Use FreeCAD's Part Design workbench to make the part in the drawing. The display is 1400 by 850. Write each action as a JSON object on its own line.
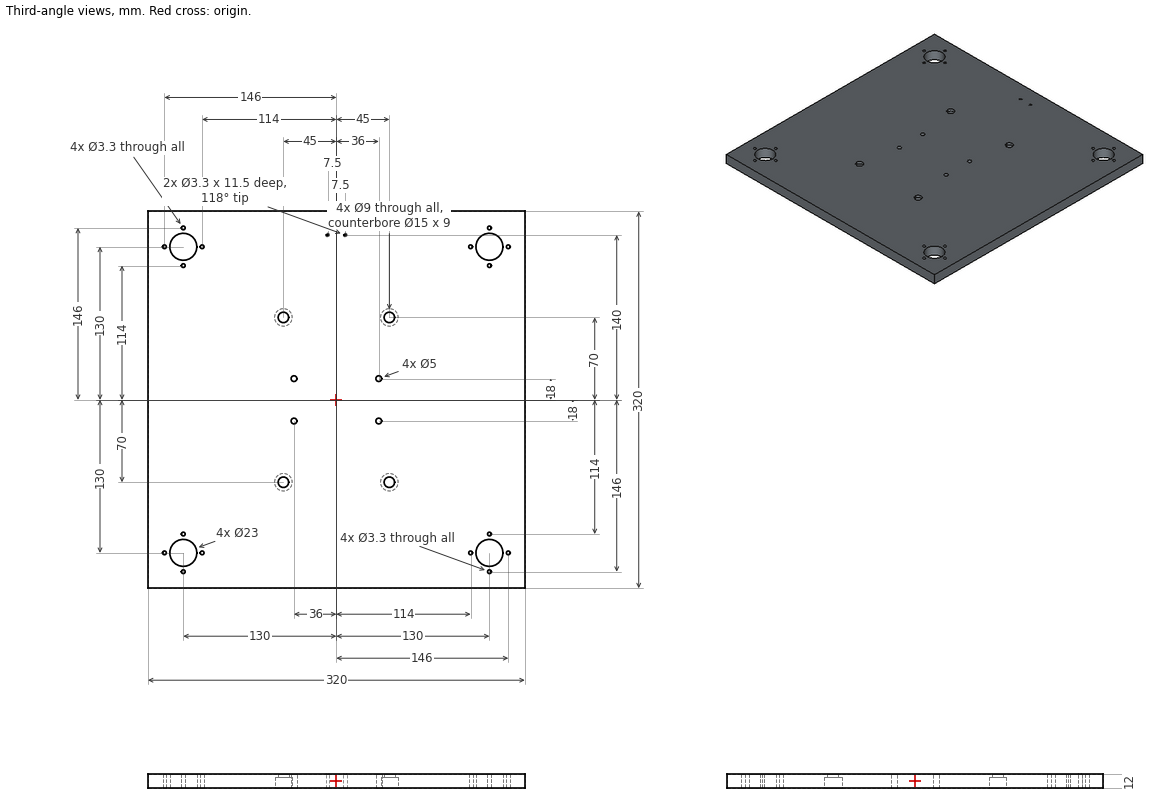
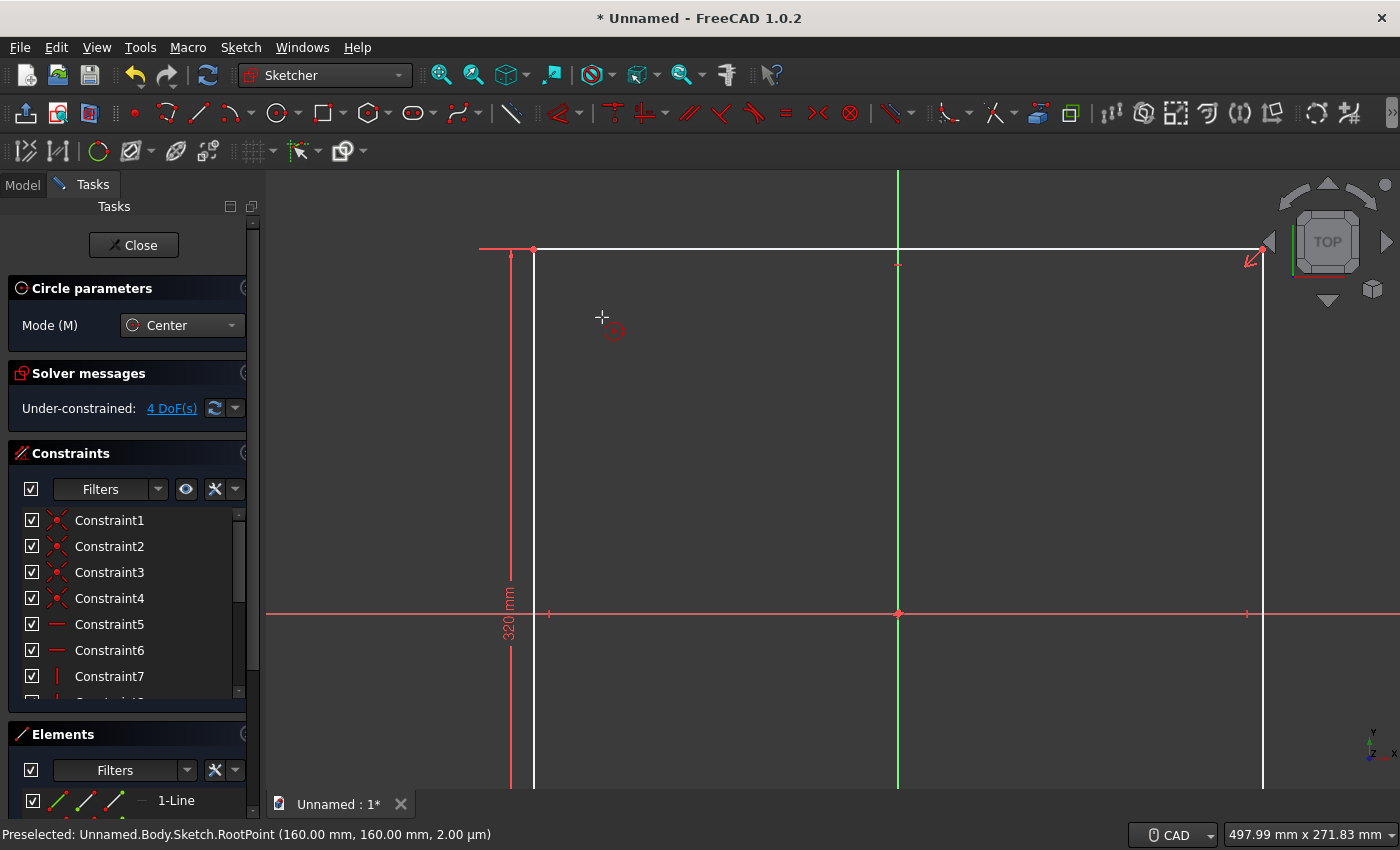
{"action": "left_click", "coordinate": [602, 317]}
{"action": "mouse_move", "coordinate": [621, 299]}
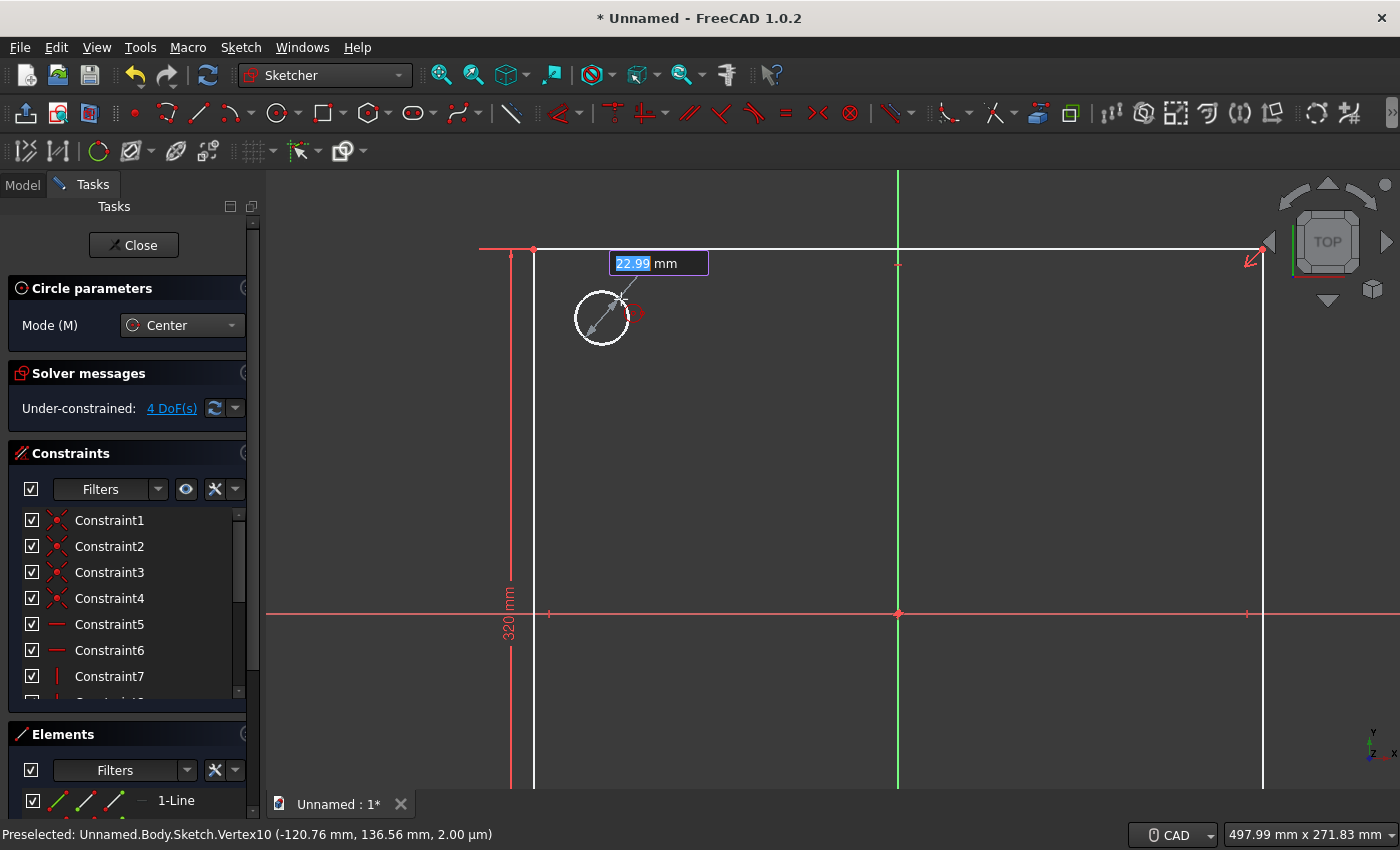
{"action": "type", "text": "23"}
{"action": "key", "text": "Return"}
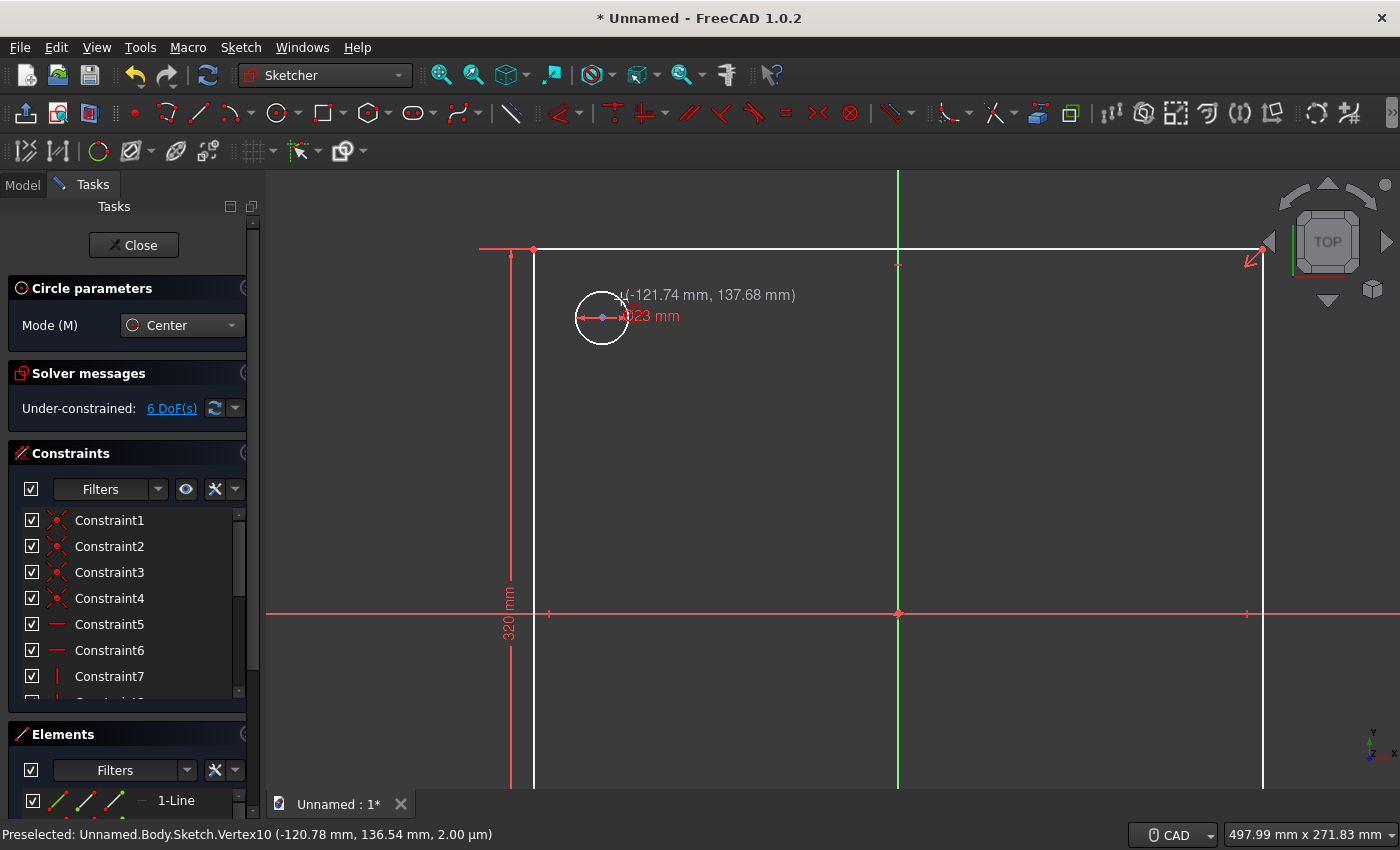
{"action": "left_click", "coordinate": [1194, 317]}
{"action": "mouse_move", "coordinate": [1213, 299]}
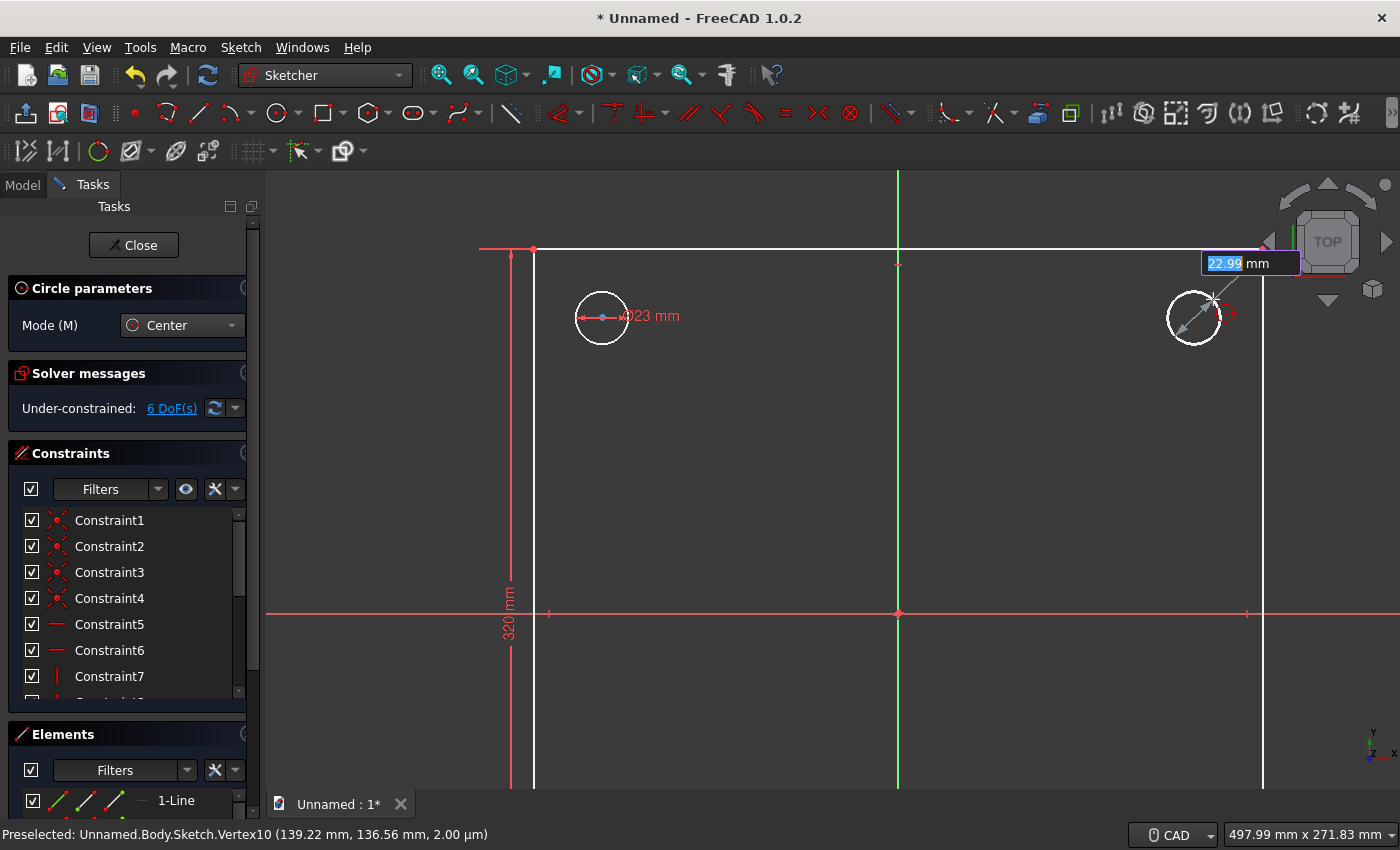
{"action": "type", "text": "23"}
{"action": "key", "text": "Return"}
{"action": "key", "text": "Escape"}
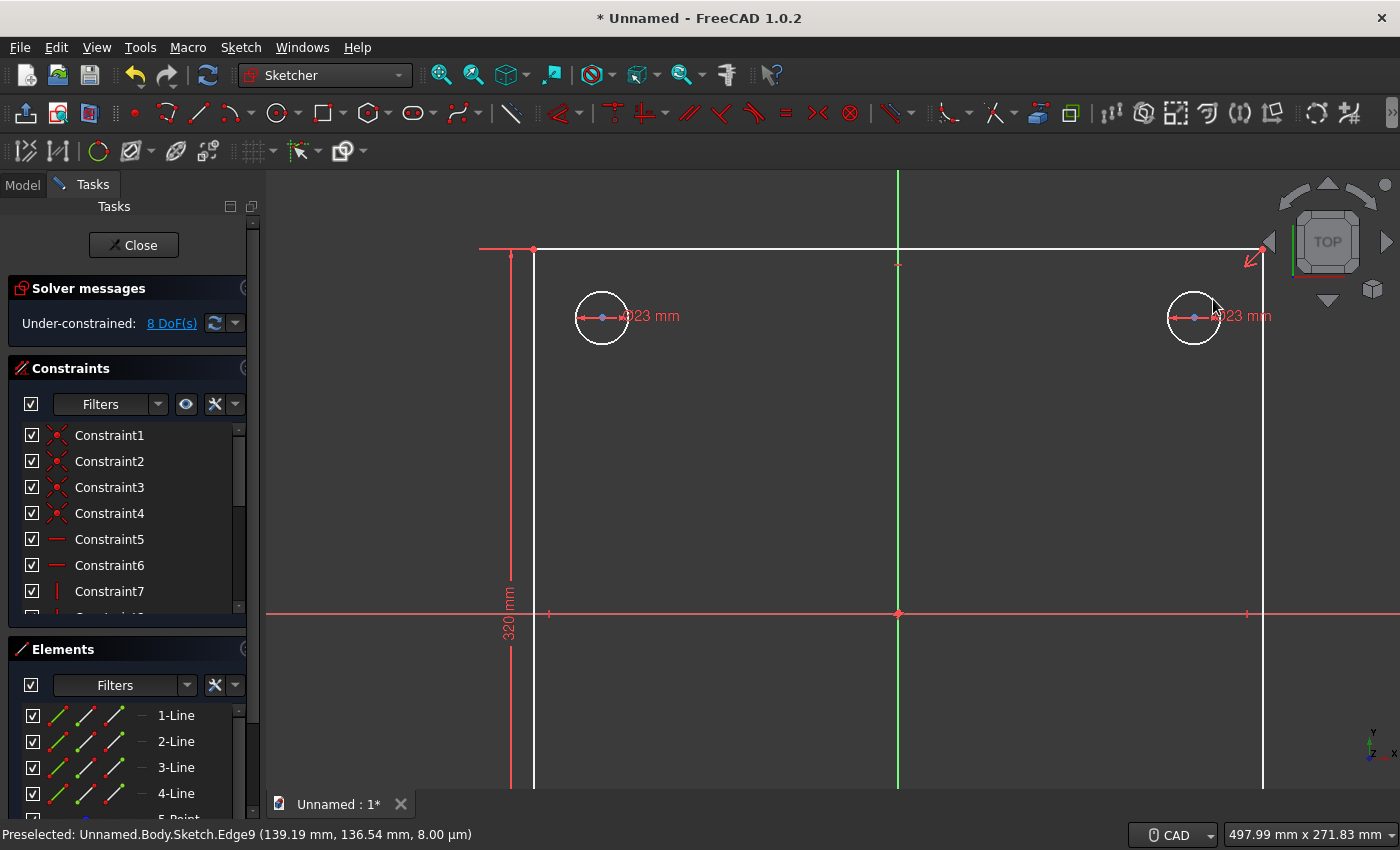
{"action": "scroll", "coordinate": [602, 316], "scroll_direction": "down", "scroll_amount": 3}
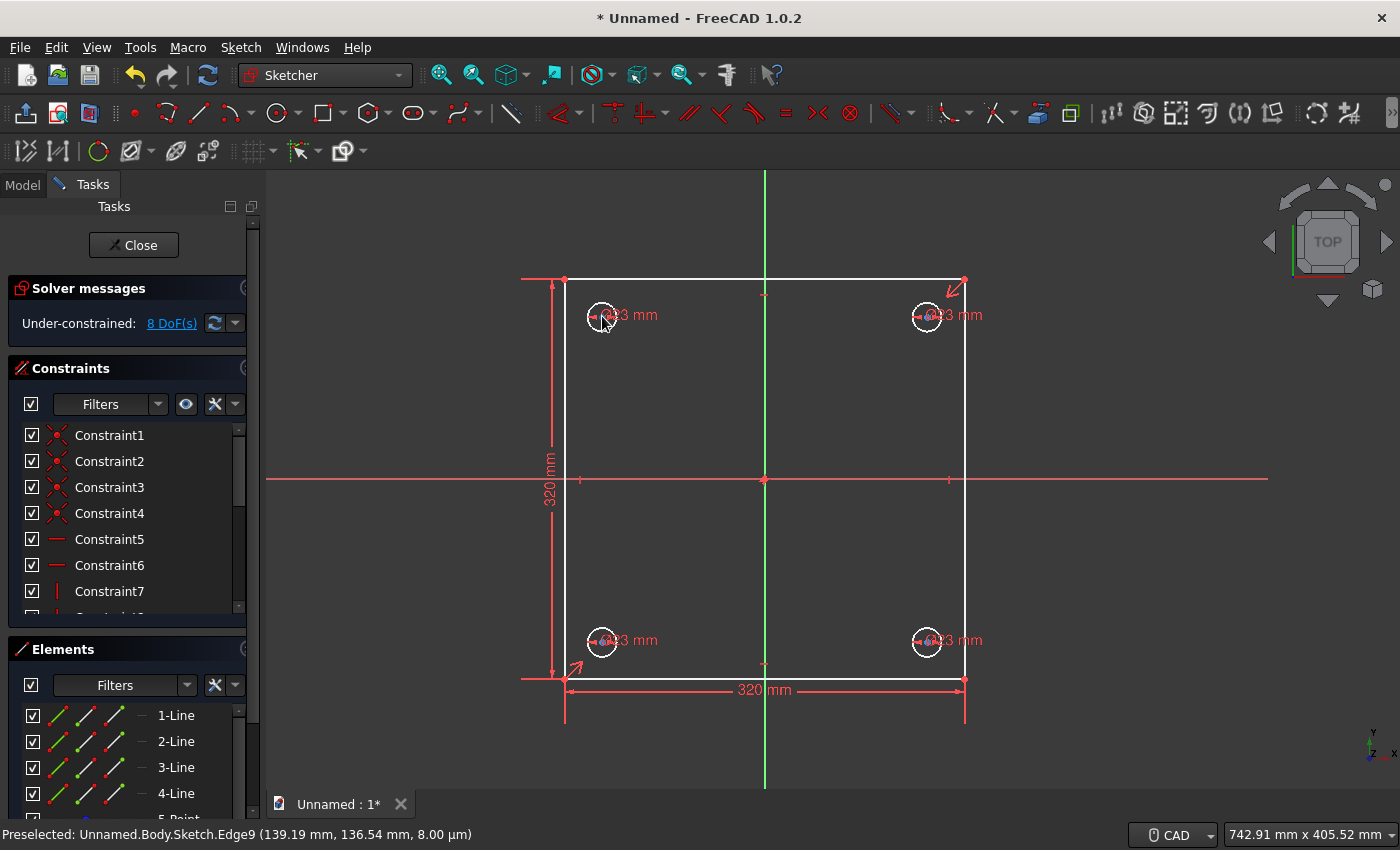
{"action": "left_click", "coordinate": [602, 642]}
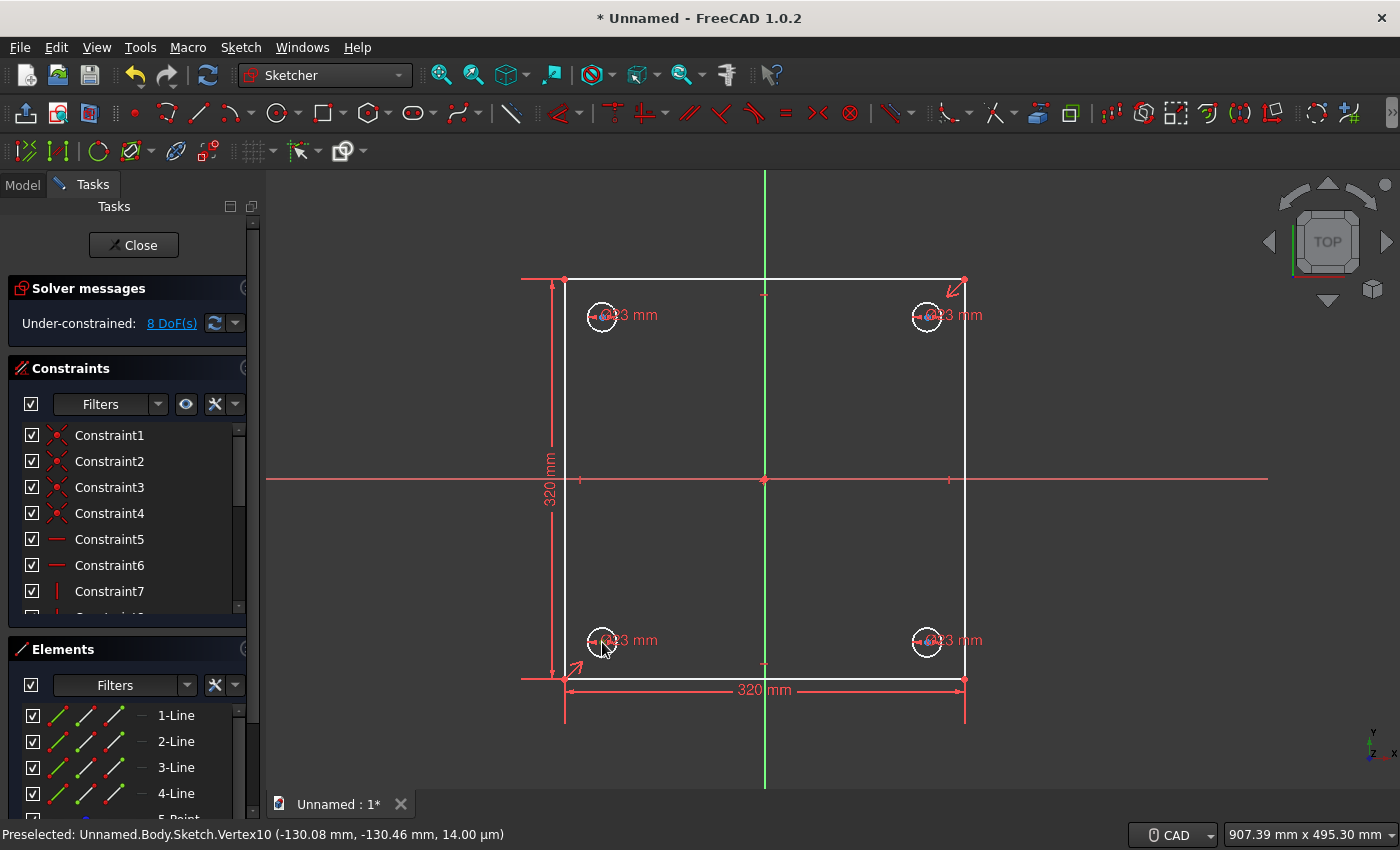
{"action": "left_click", "coordinate": [927, 642]}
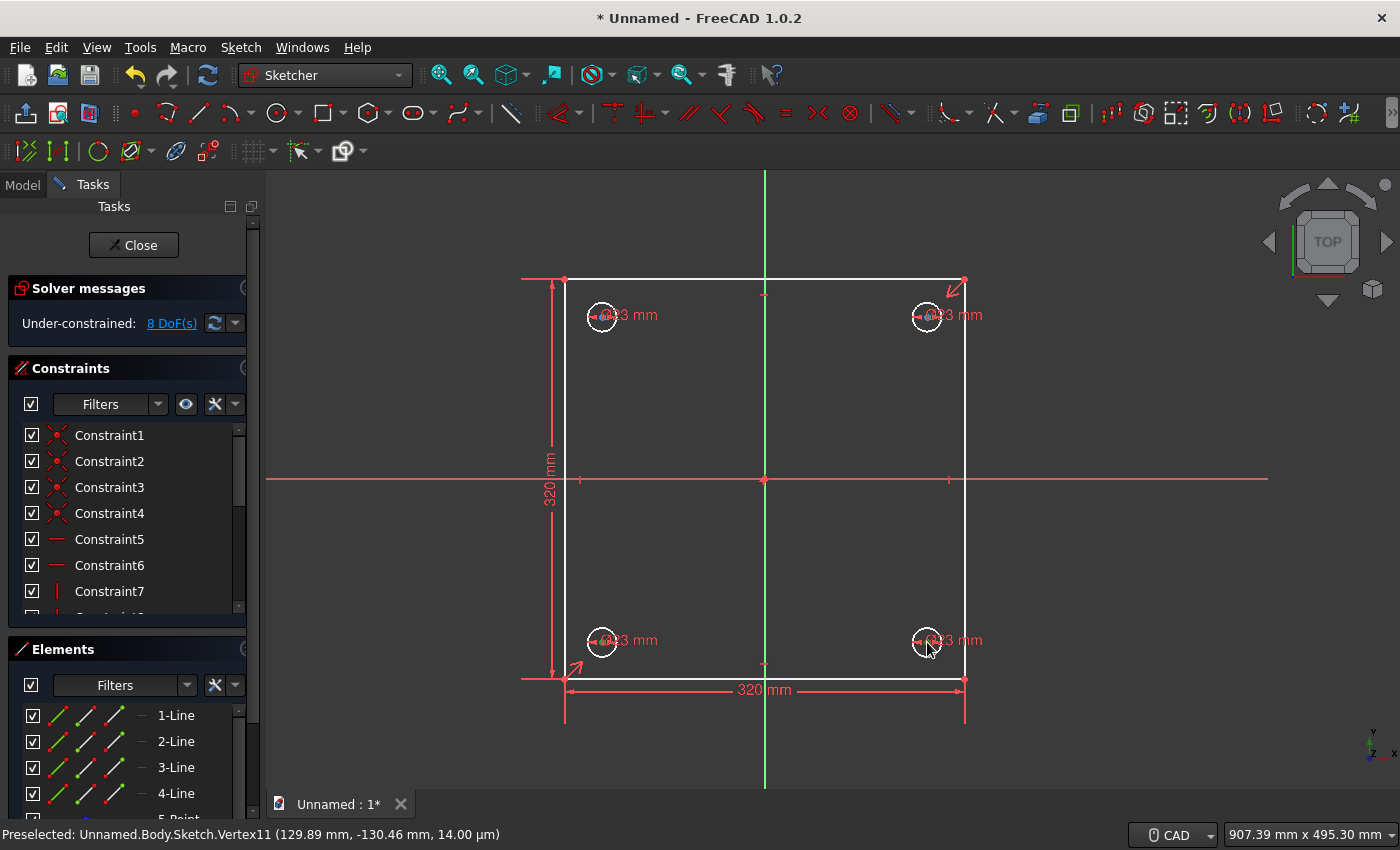
{"action": "key", "text": "h"}